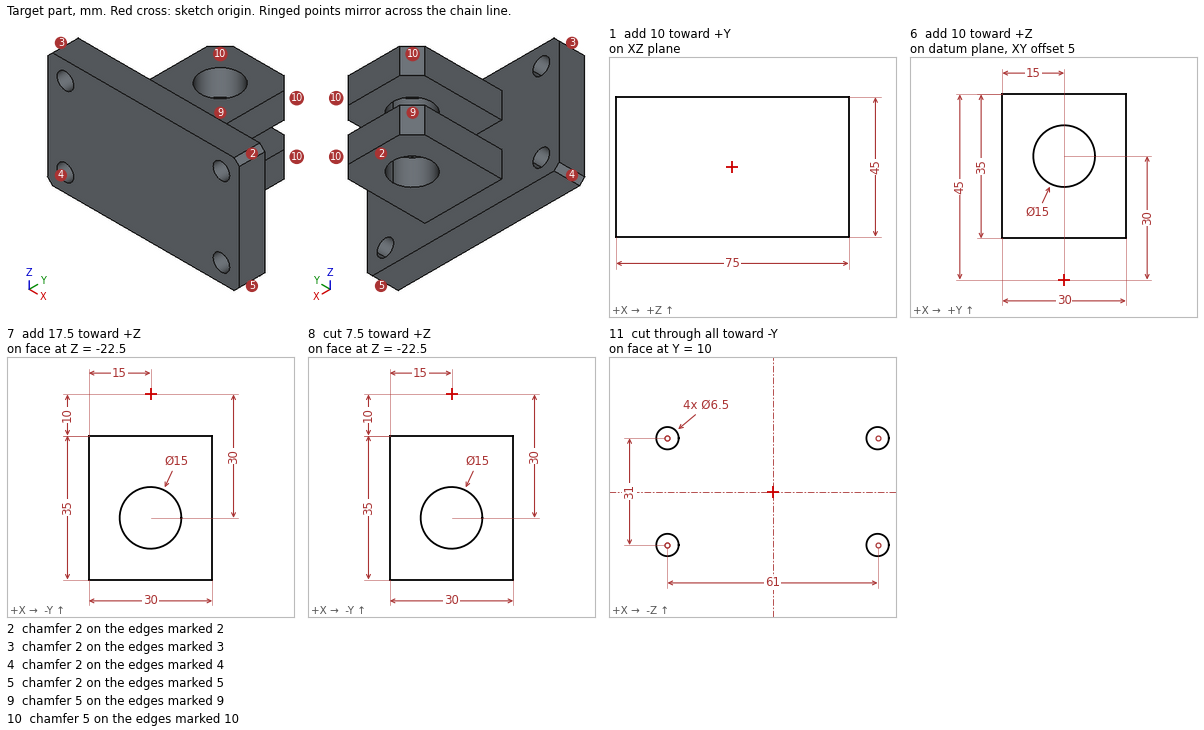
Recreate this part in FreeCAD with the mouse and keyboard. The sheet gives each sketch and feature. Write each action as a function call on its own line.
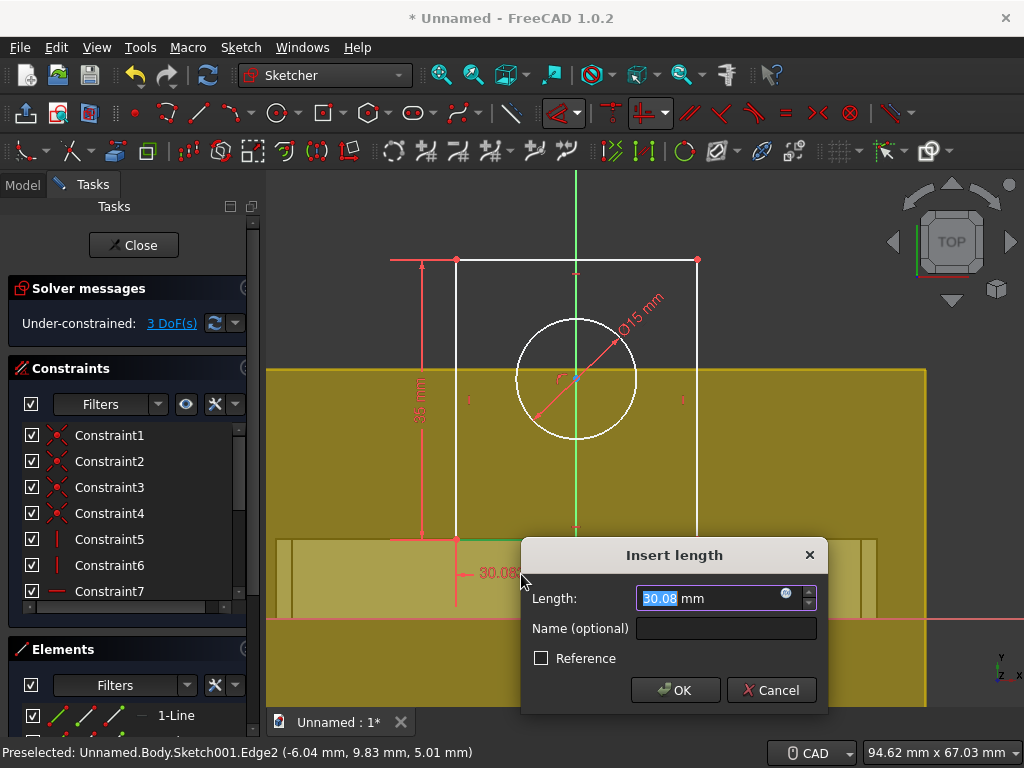
text(30)
key(Return)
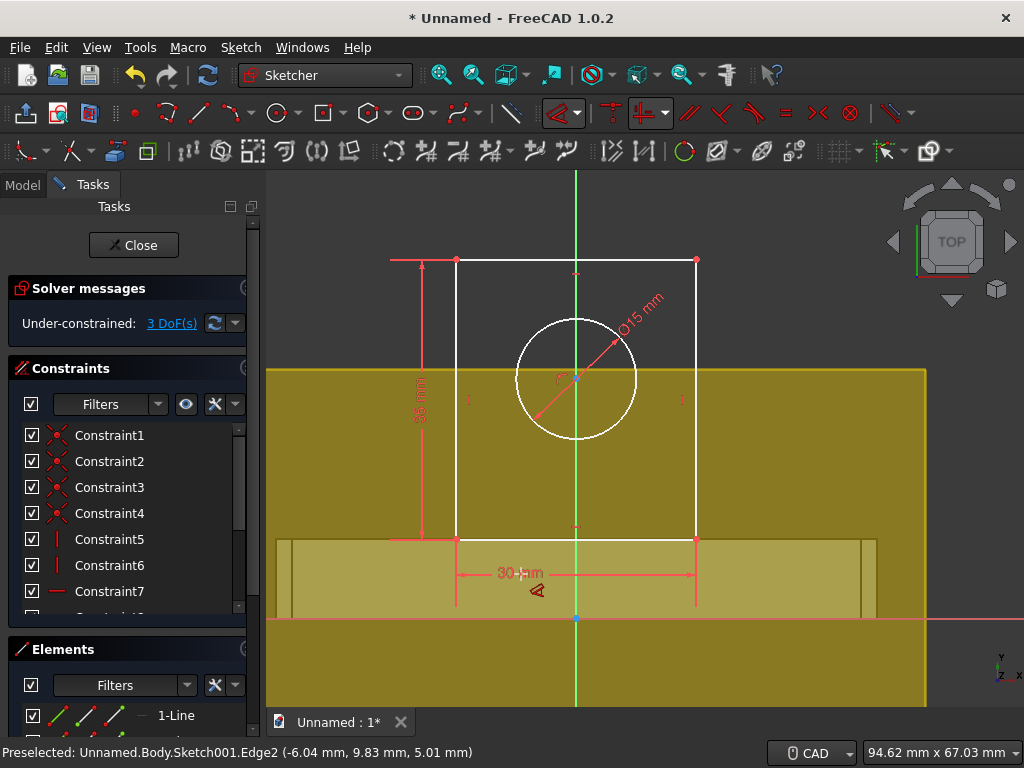
click(576, 379)
click(610, 499)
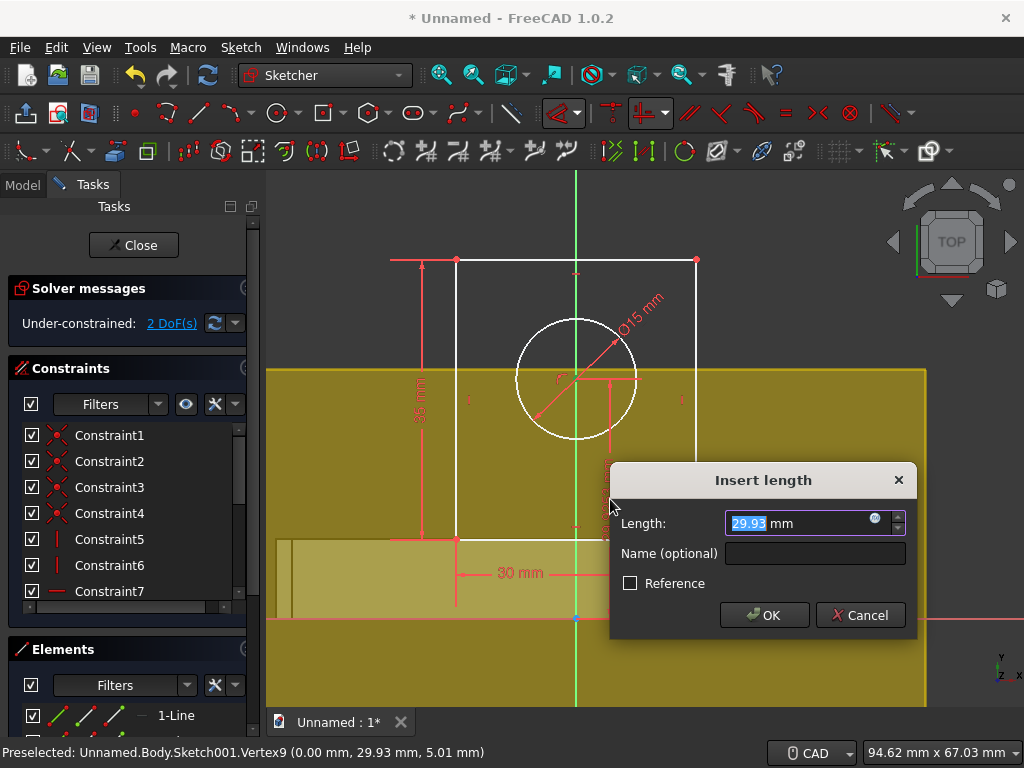
text(30)
key(Return)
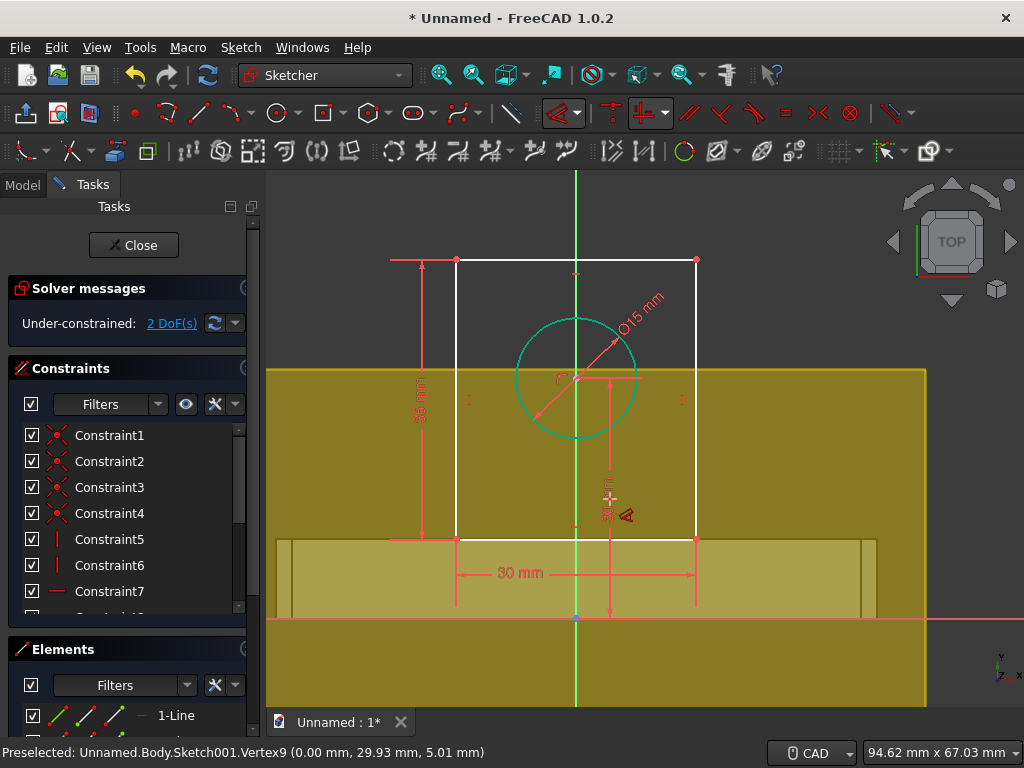
click(456, 260)
click(516, 653)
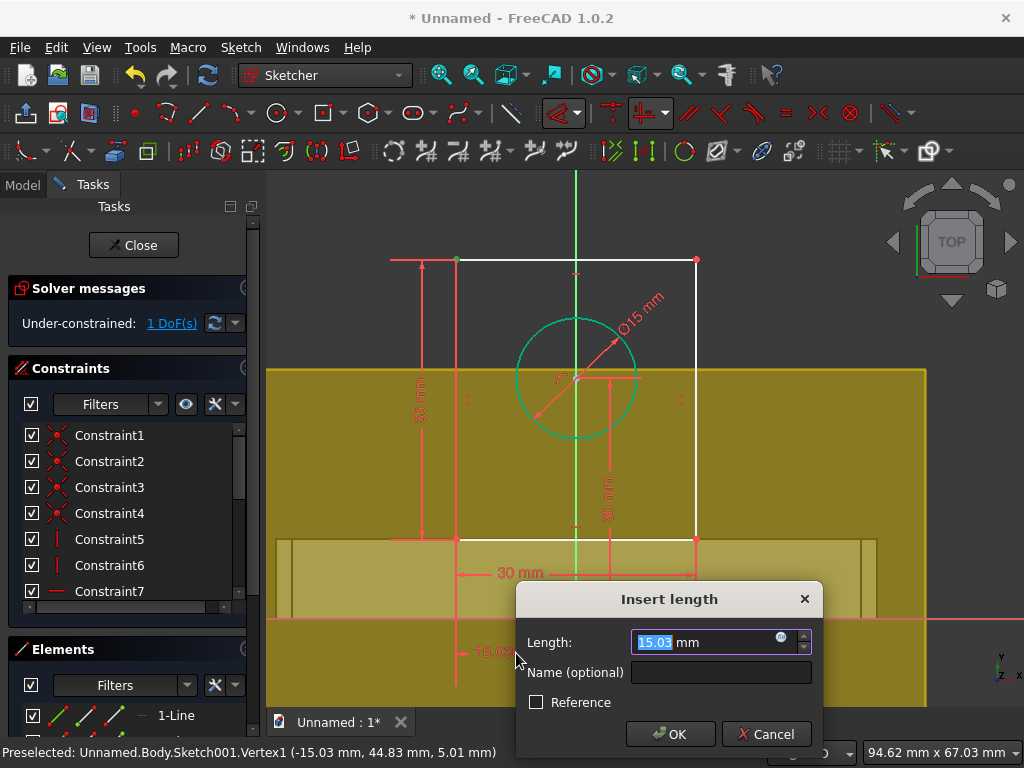
text(15)
key(Return)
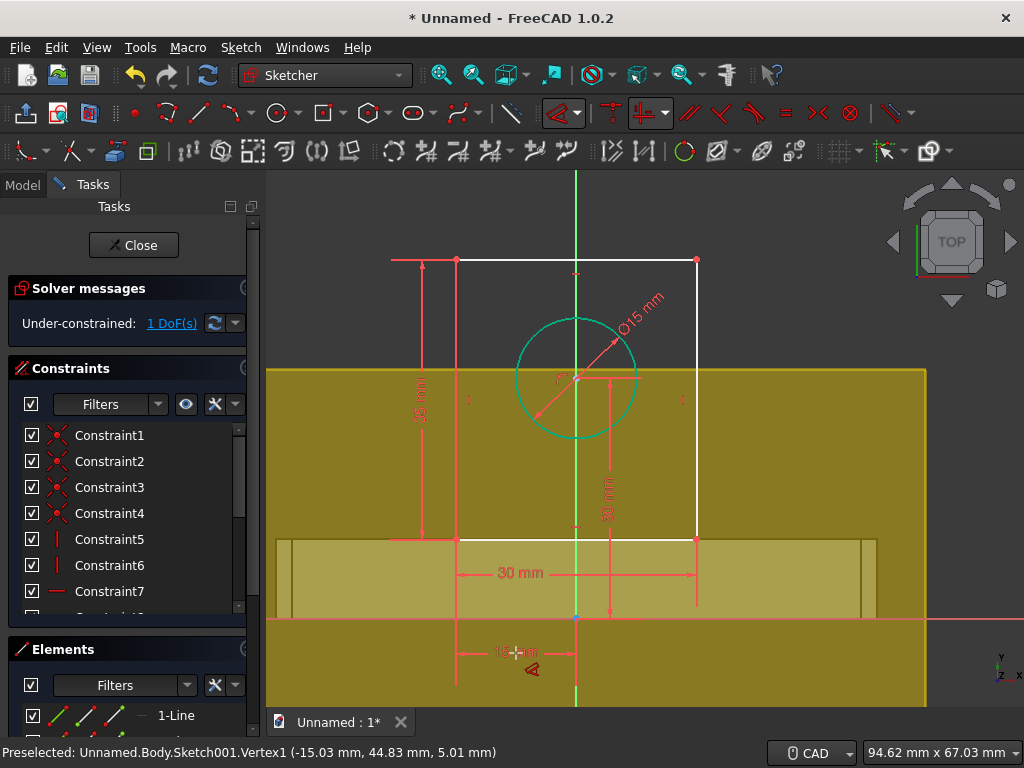
click(456, 260)
click(422, 439)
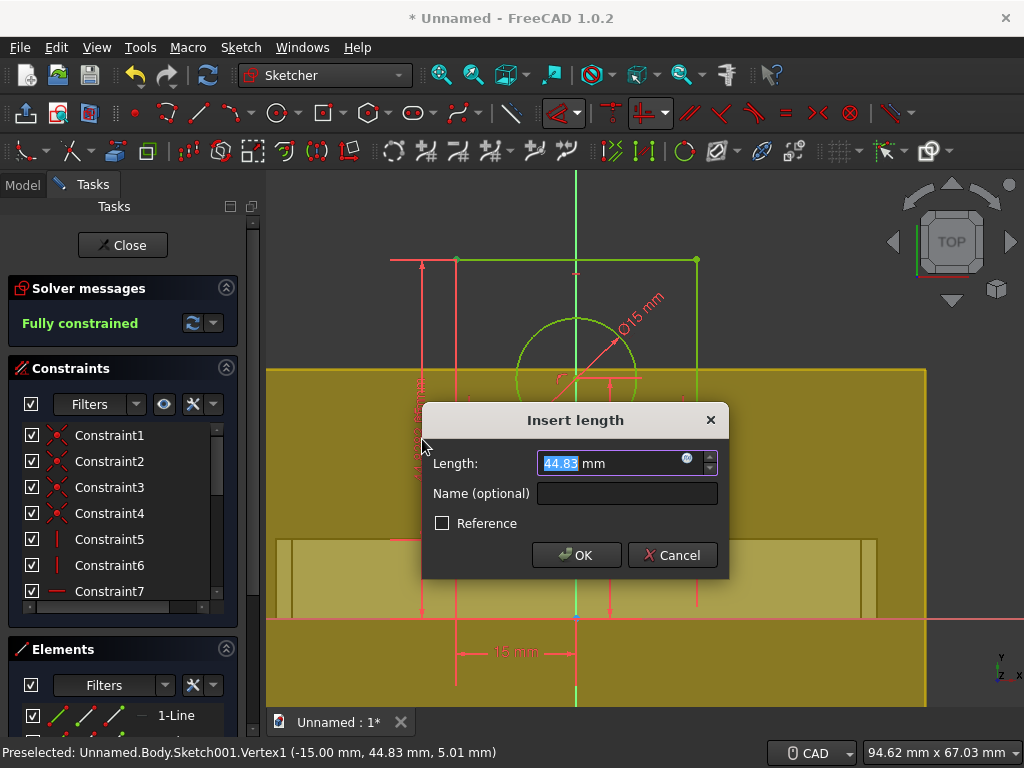
text(45)
key(Return)
key(Escape)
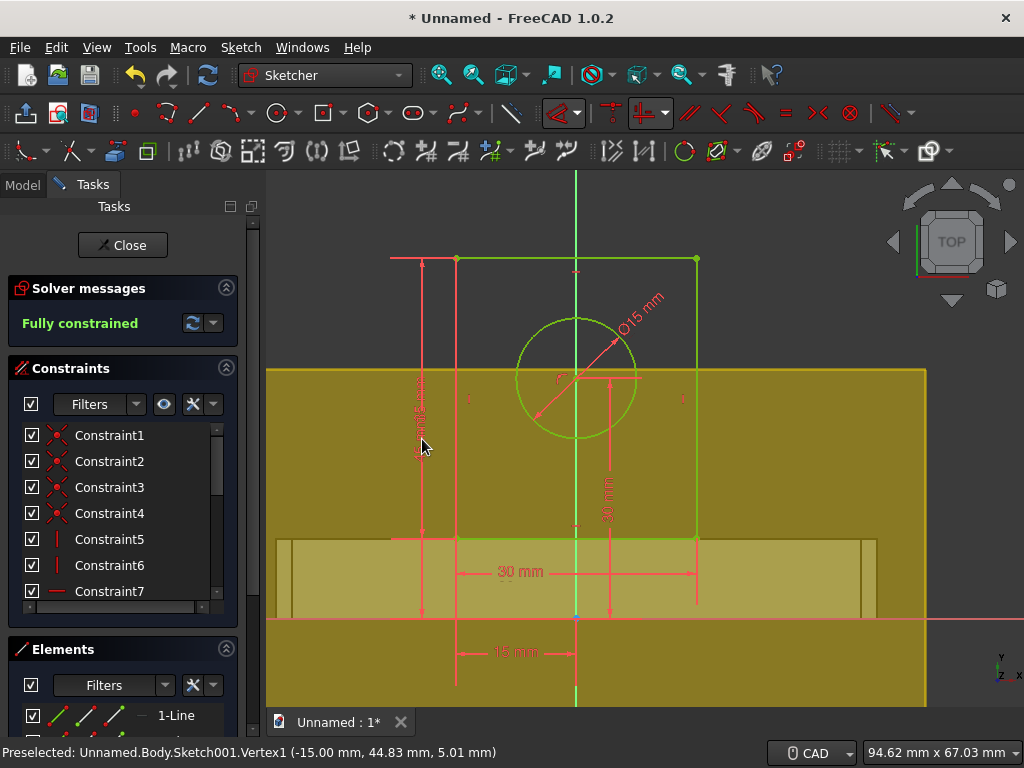
click(123, 245)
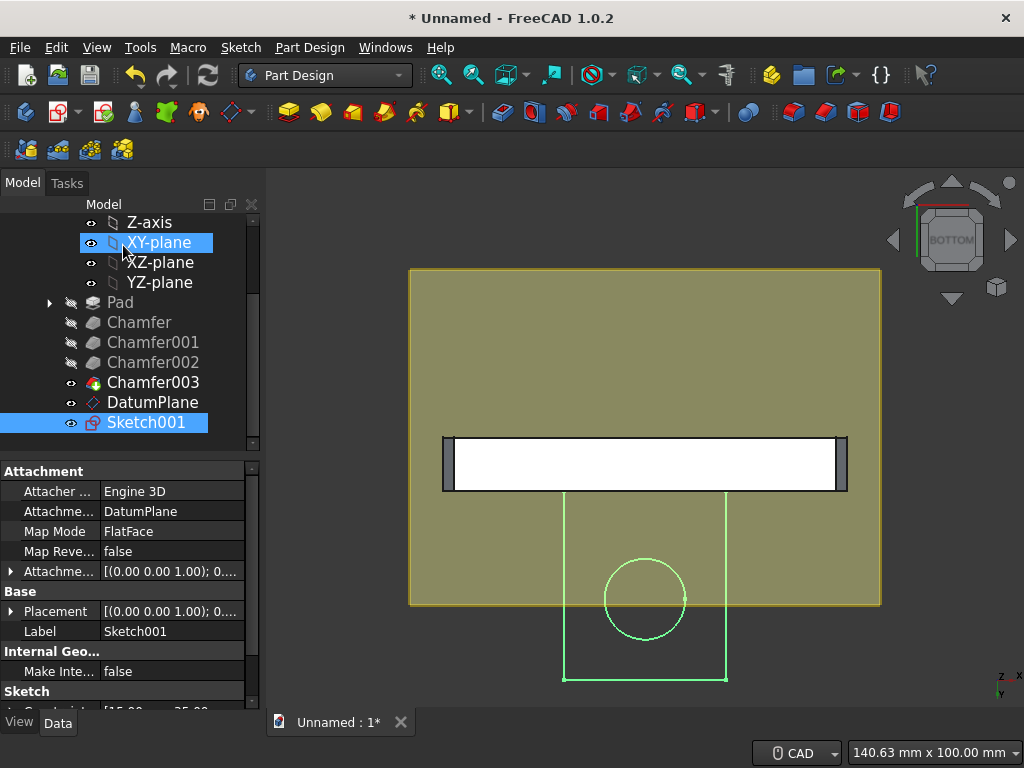
click(290, 112)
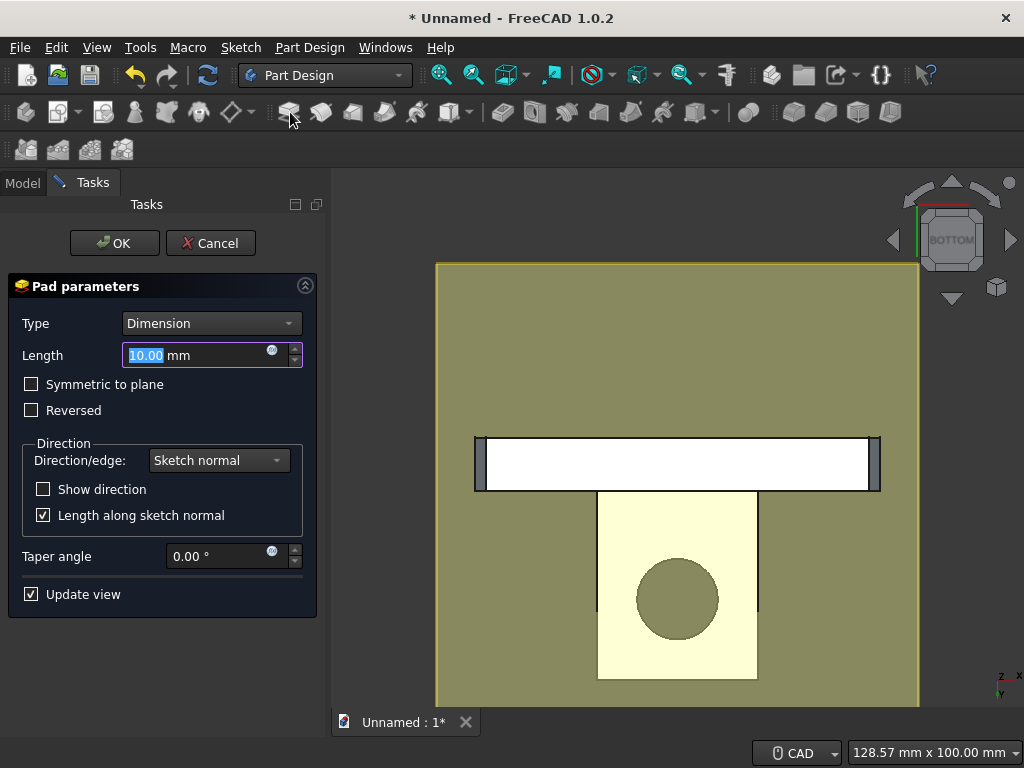
text(10)
key(Tab)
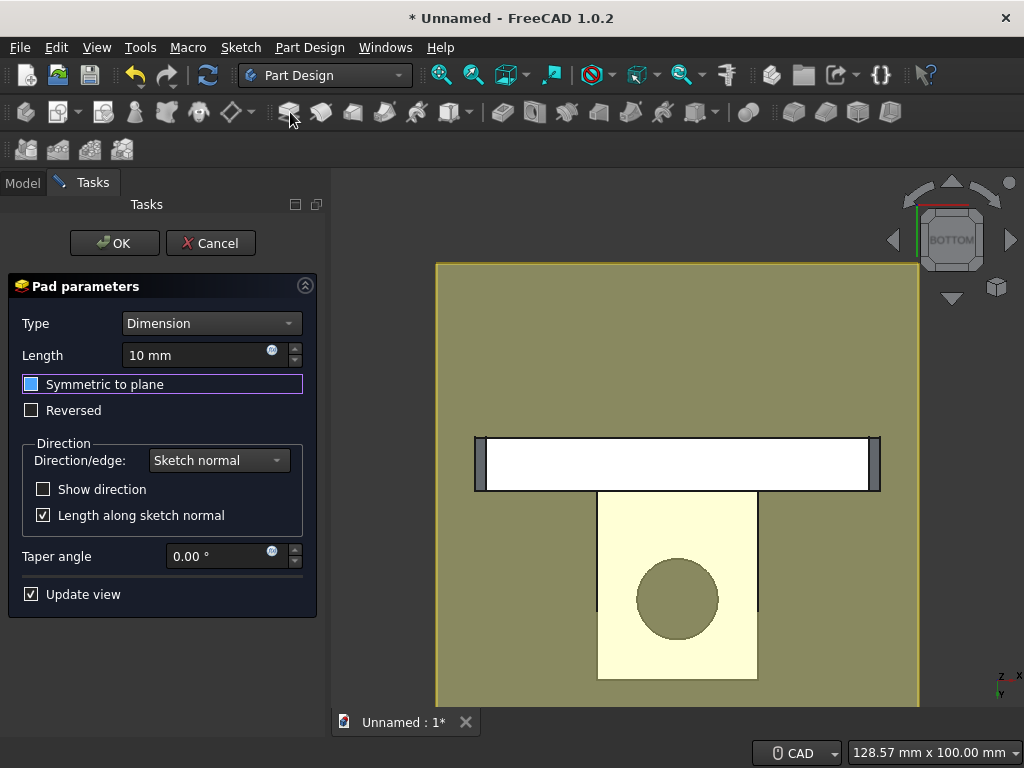
click(115, 243)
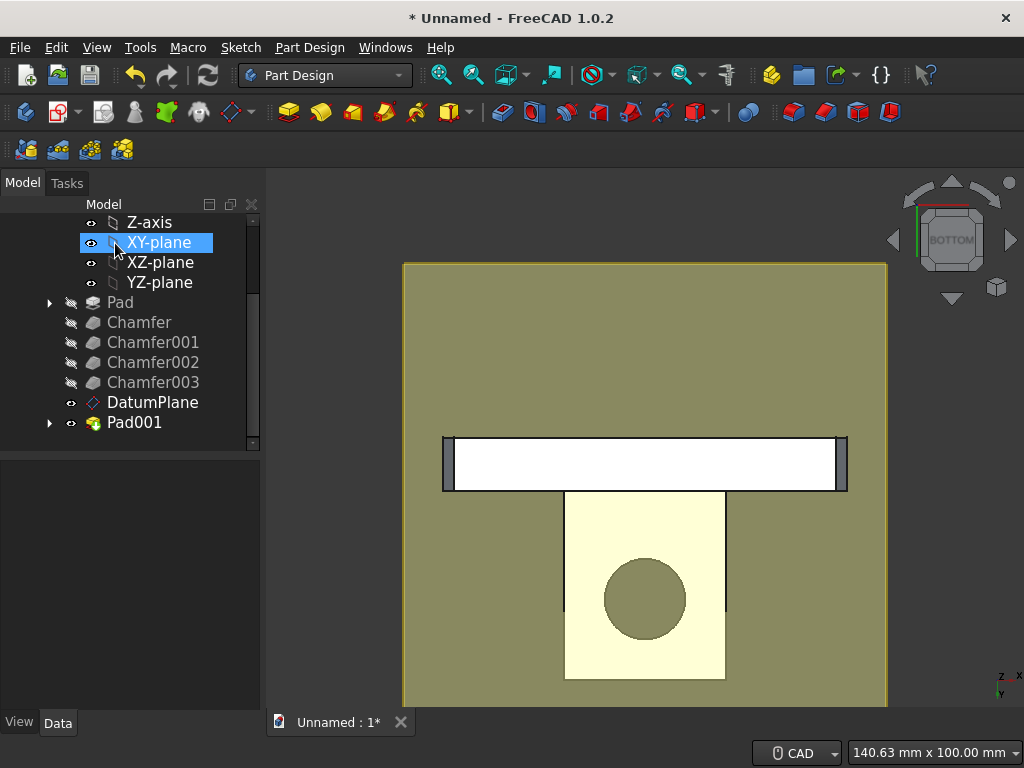
click(116, 403)
key(space)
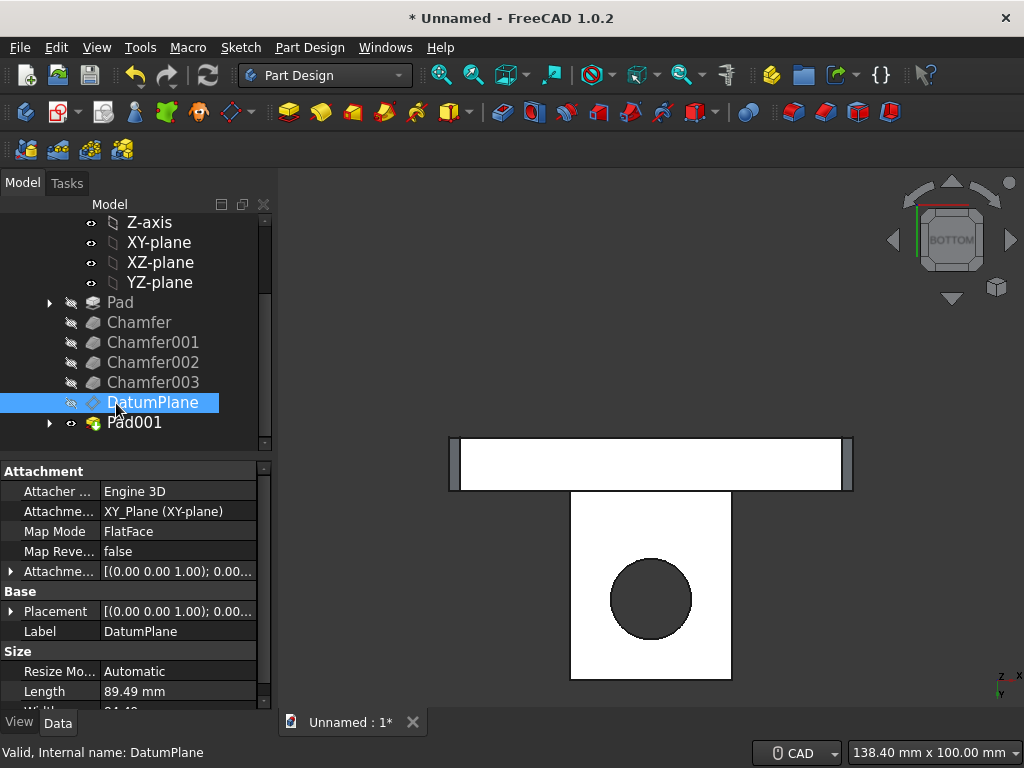
click(815, 463)